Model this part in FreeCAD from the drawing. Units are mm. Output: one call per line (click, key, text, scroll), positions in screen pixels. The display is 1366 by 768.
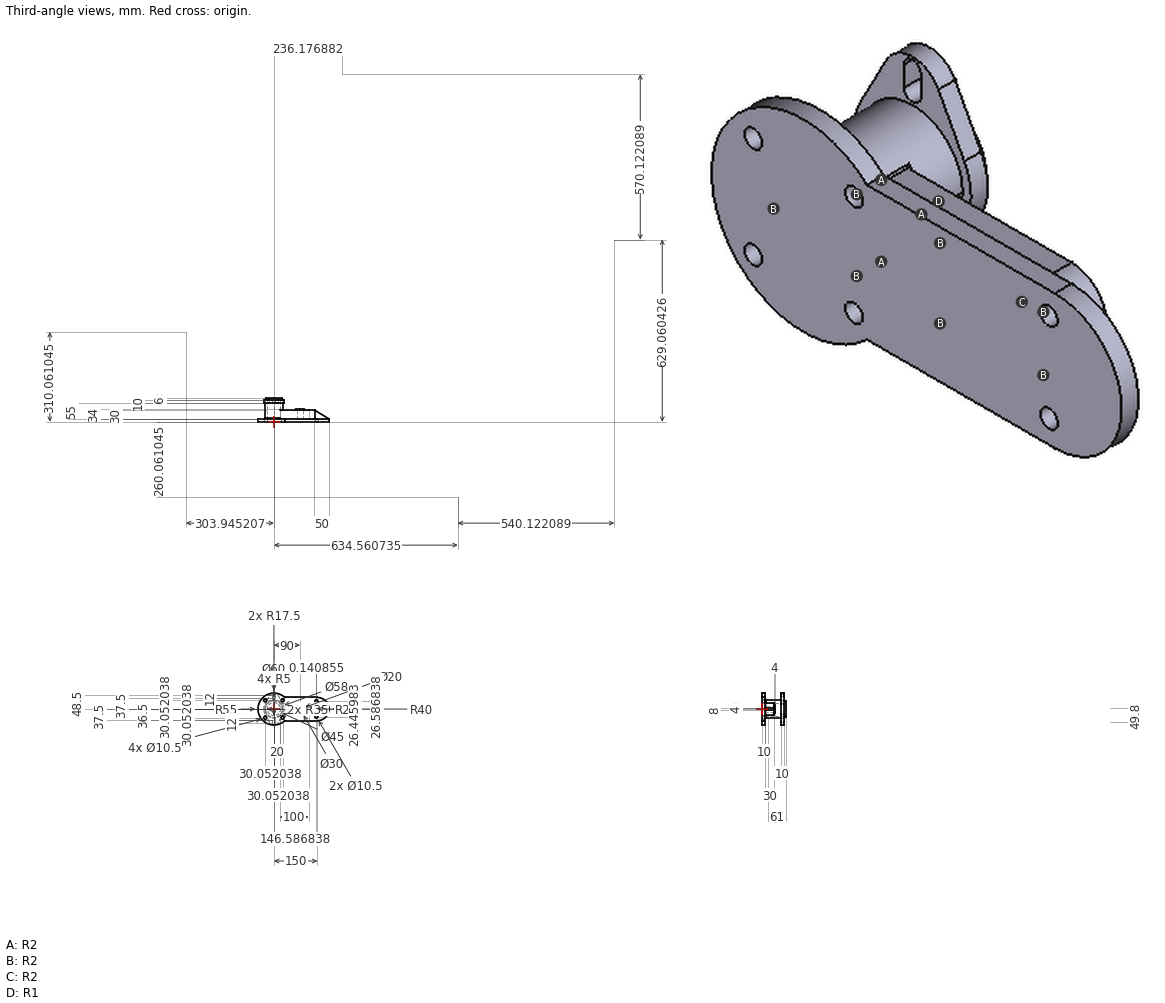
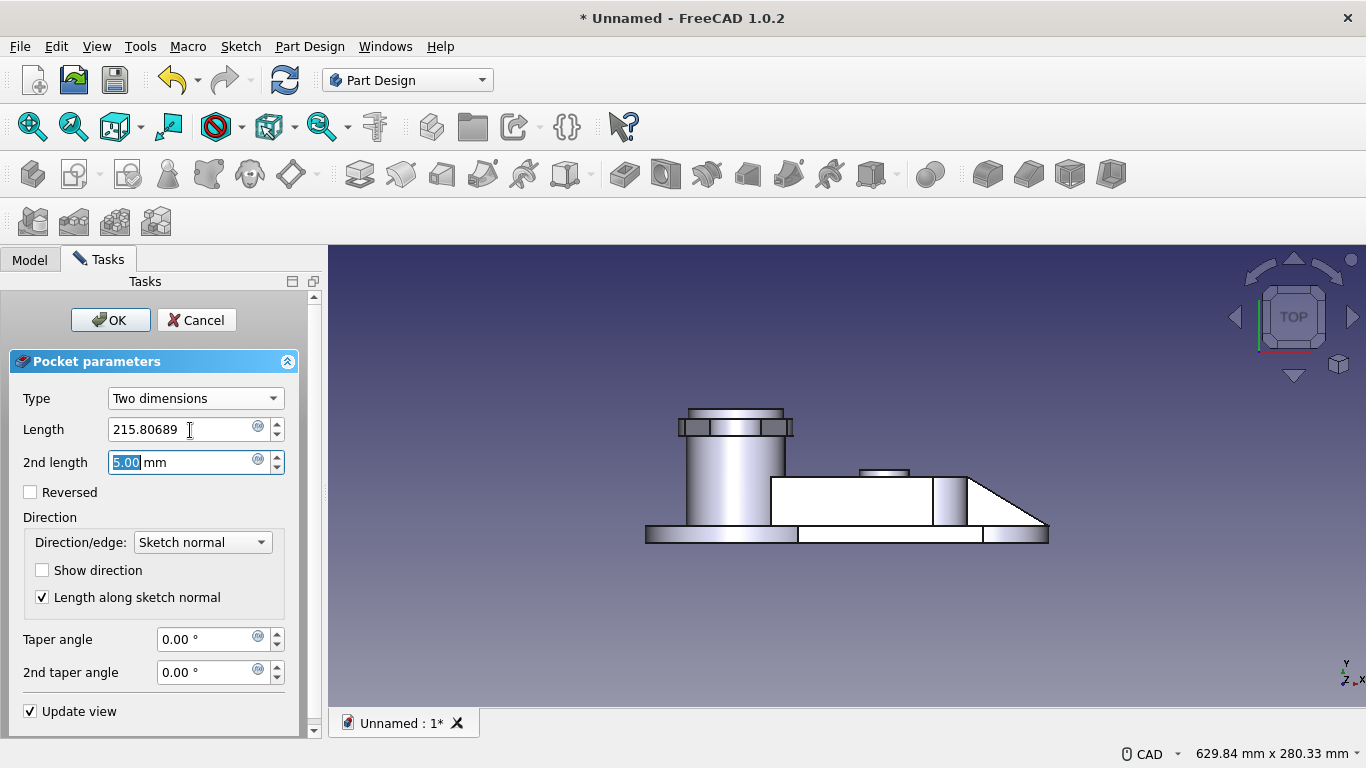
text(49.8)
key(Tab)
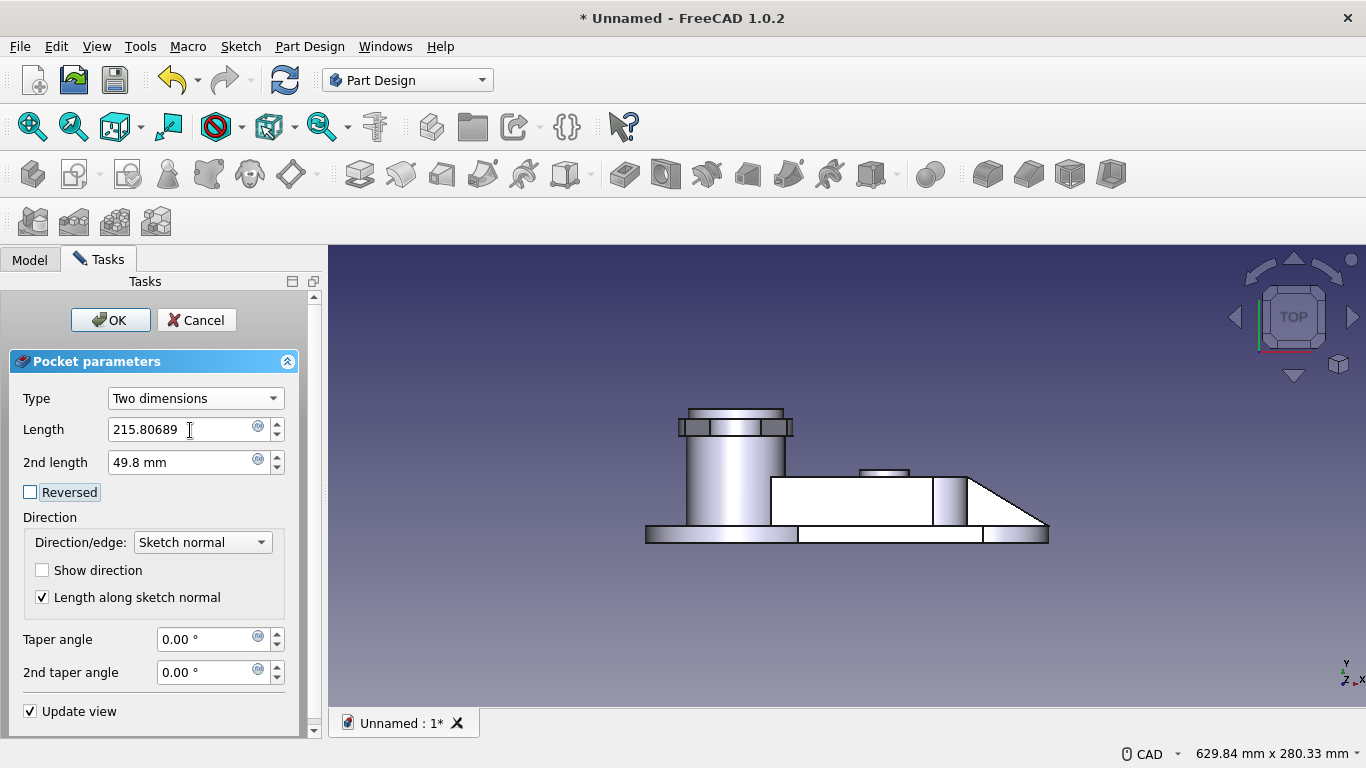
click(31, 492)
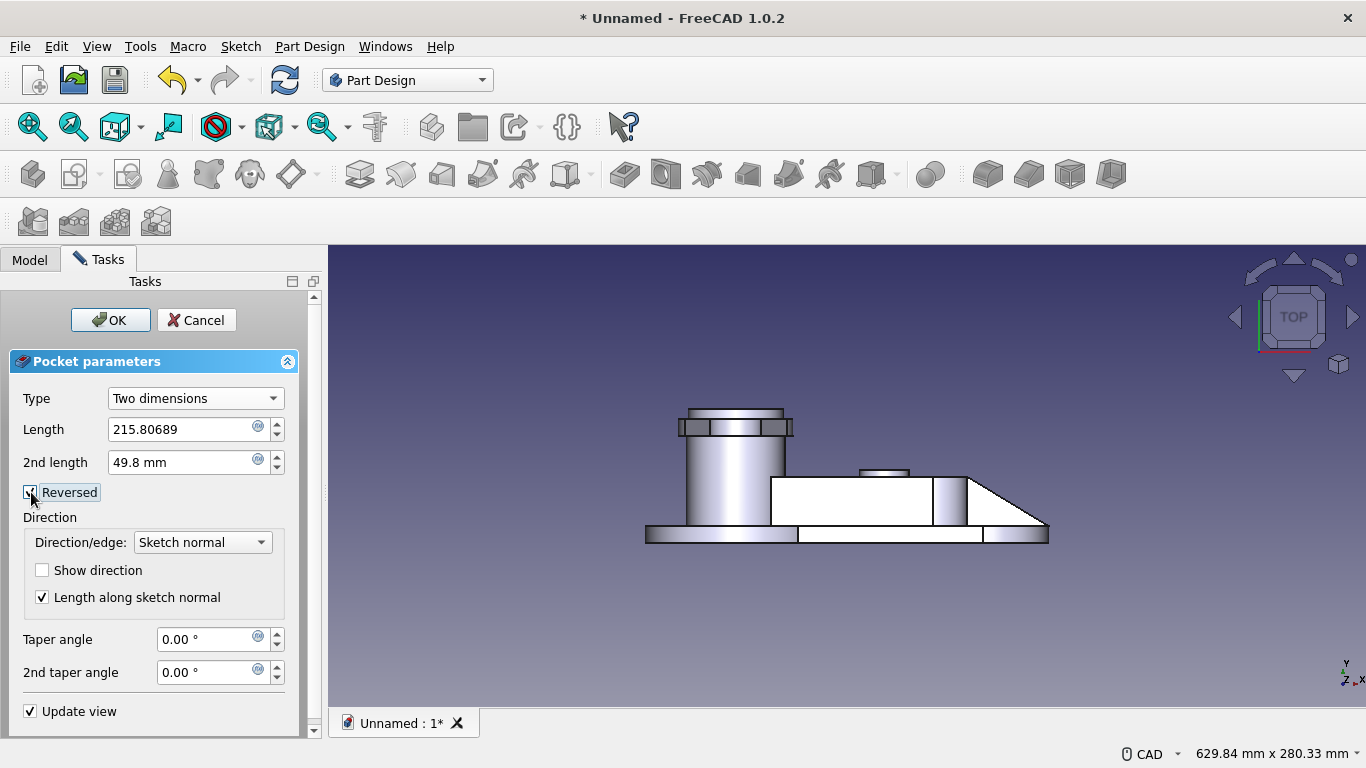
click(111, 320)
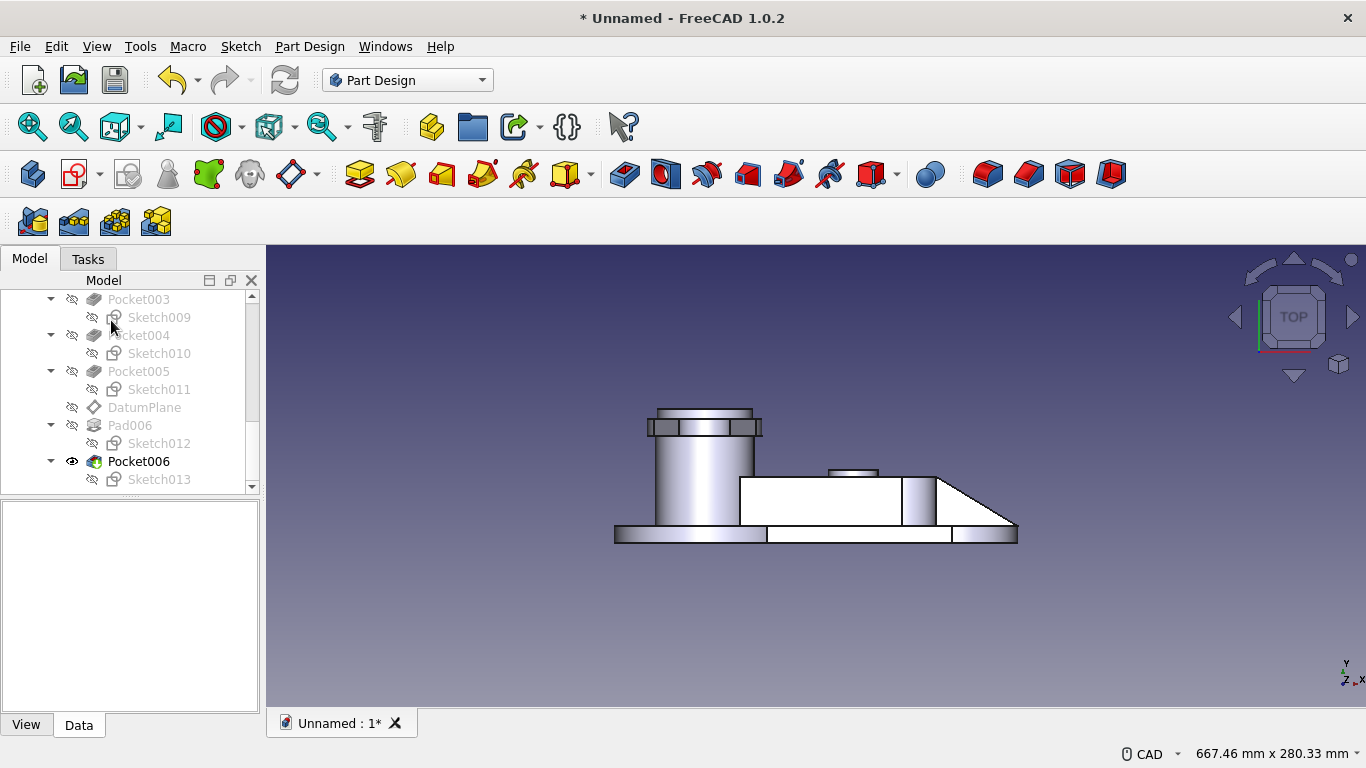
click(33, 128)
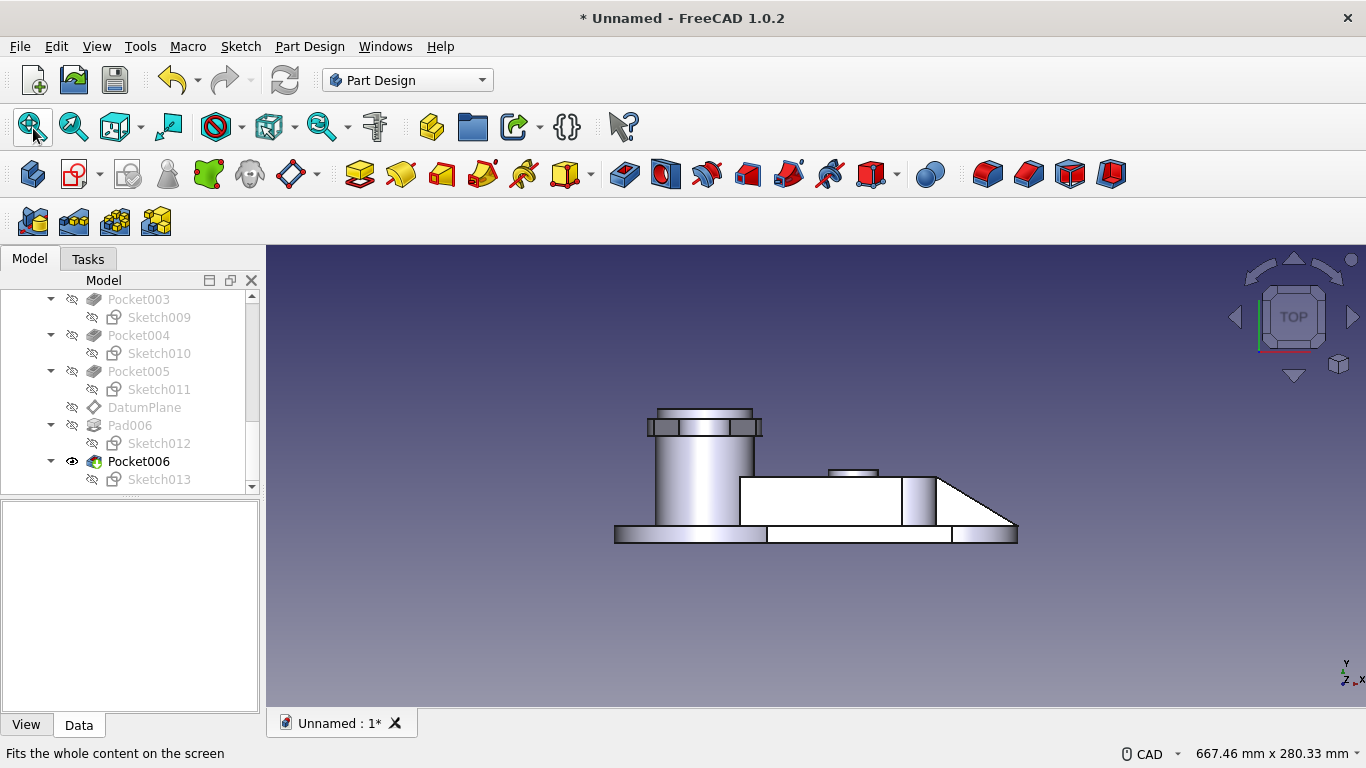
key(0)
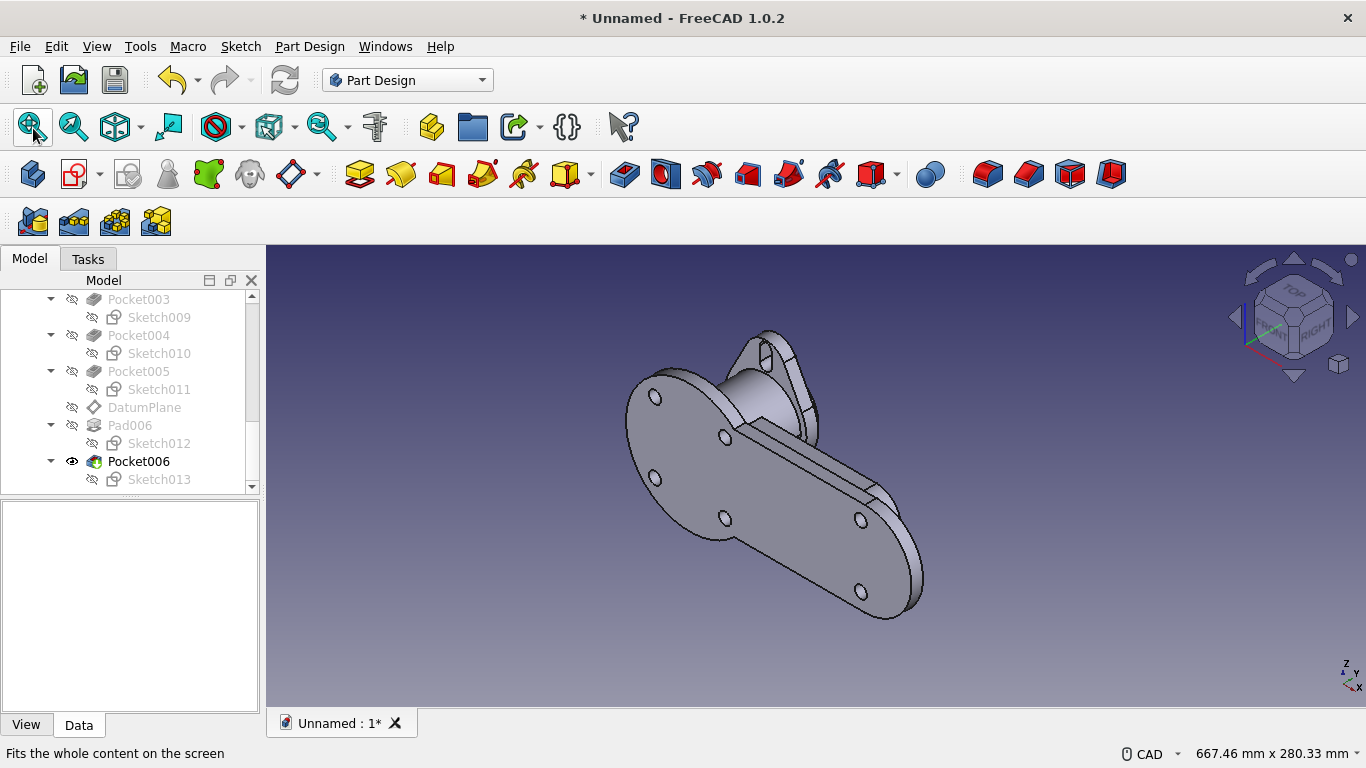
key(2)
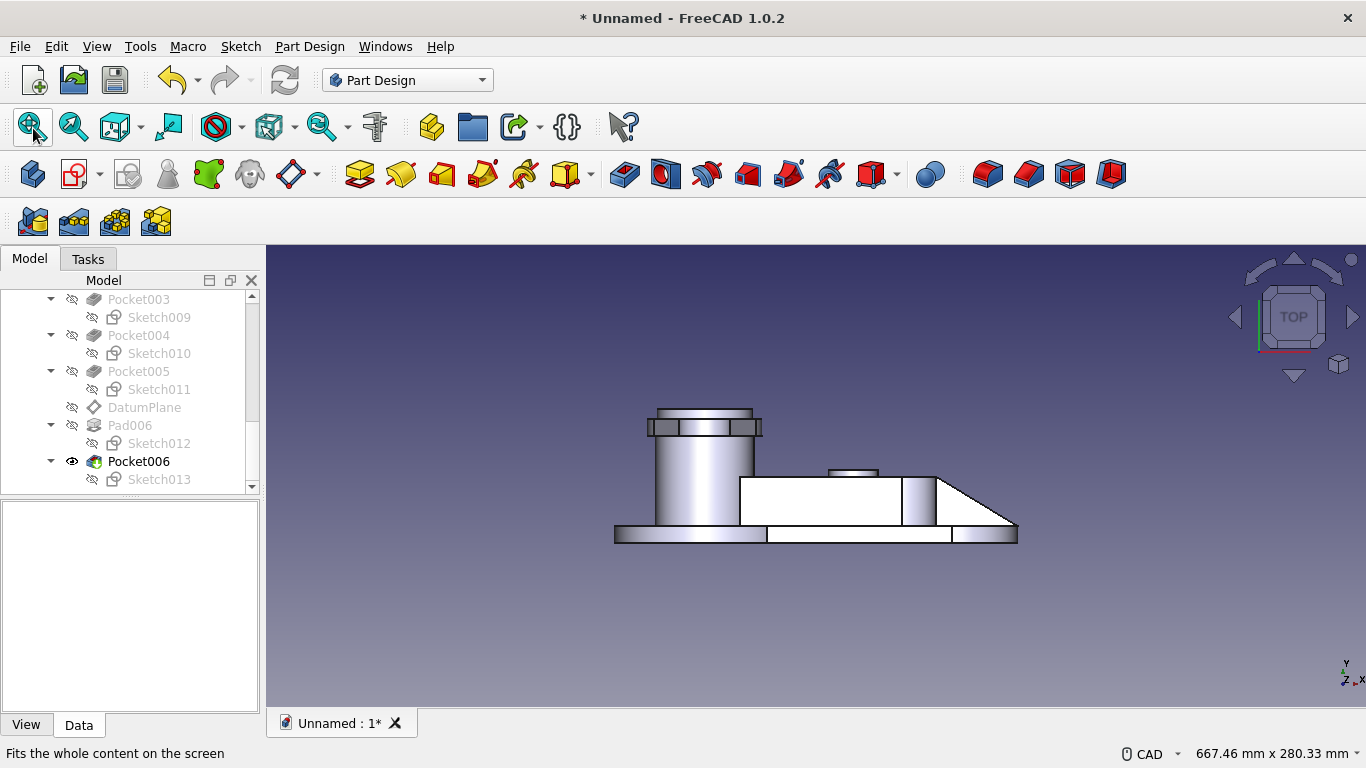
key(v)
key(f)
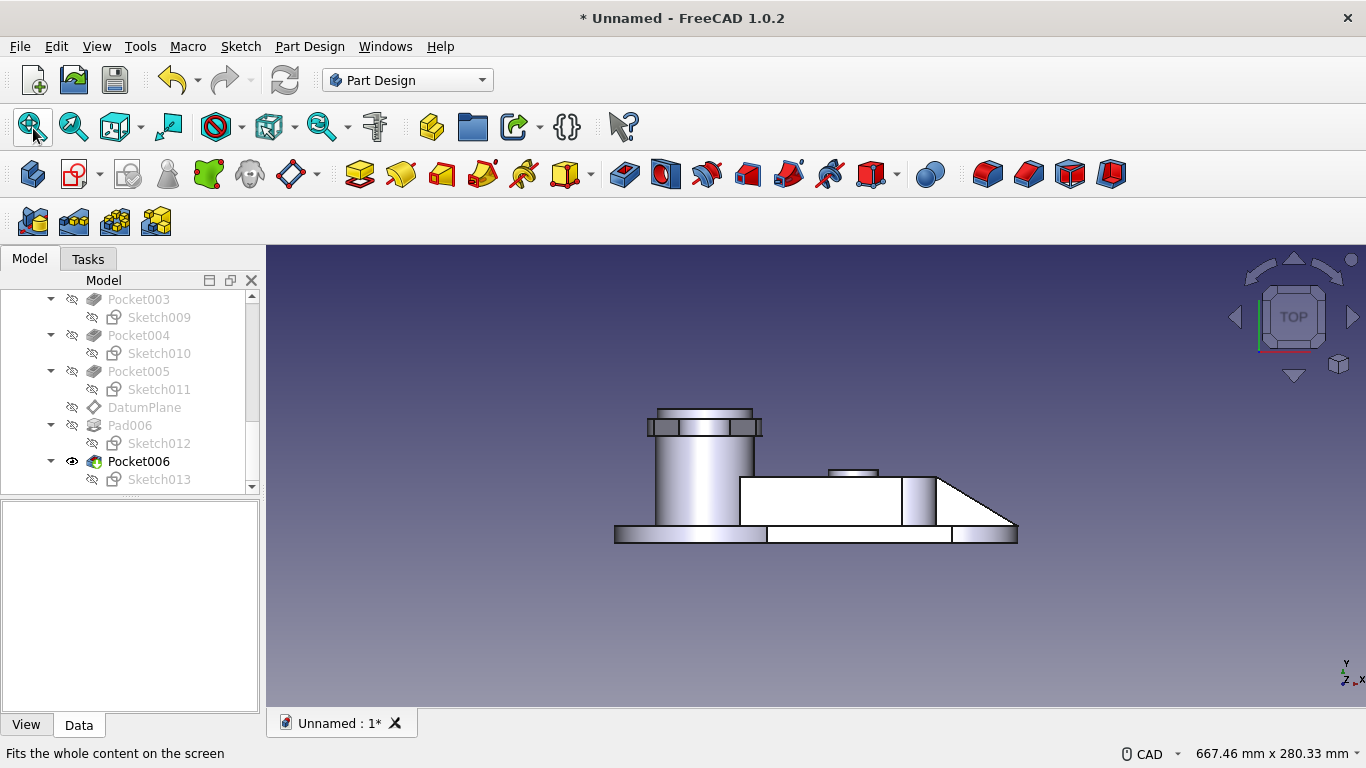
key(1)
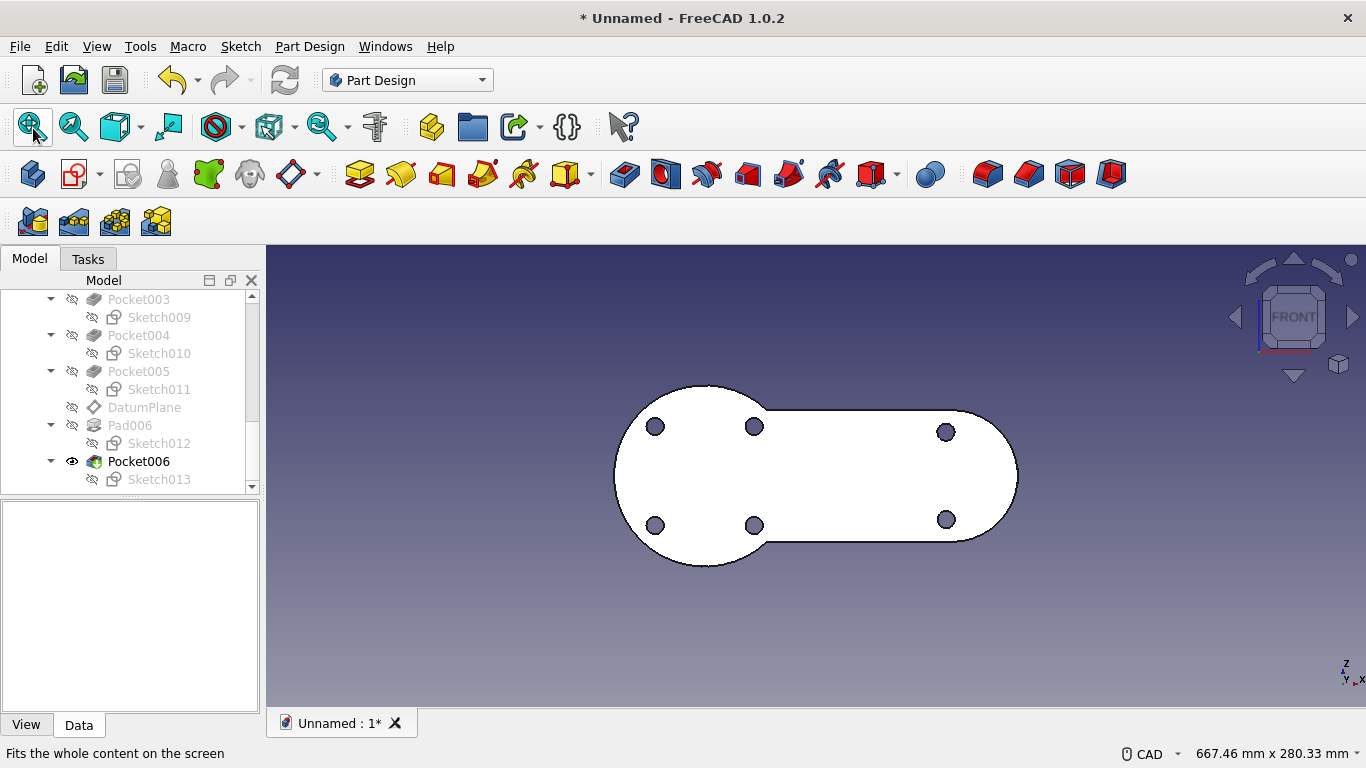
click(33, 128)